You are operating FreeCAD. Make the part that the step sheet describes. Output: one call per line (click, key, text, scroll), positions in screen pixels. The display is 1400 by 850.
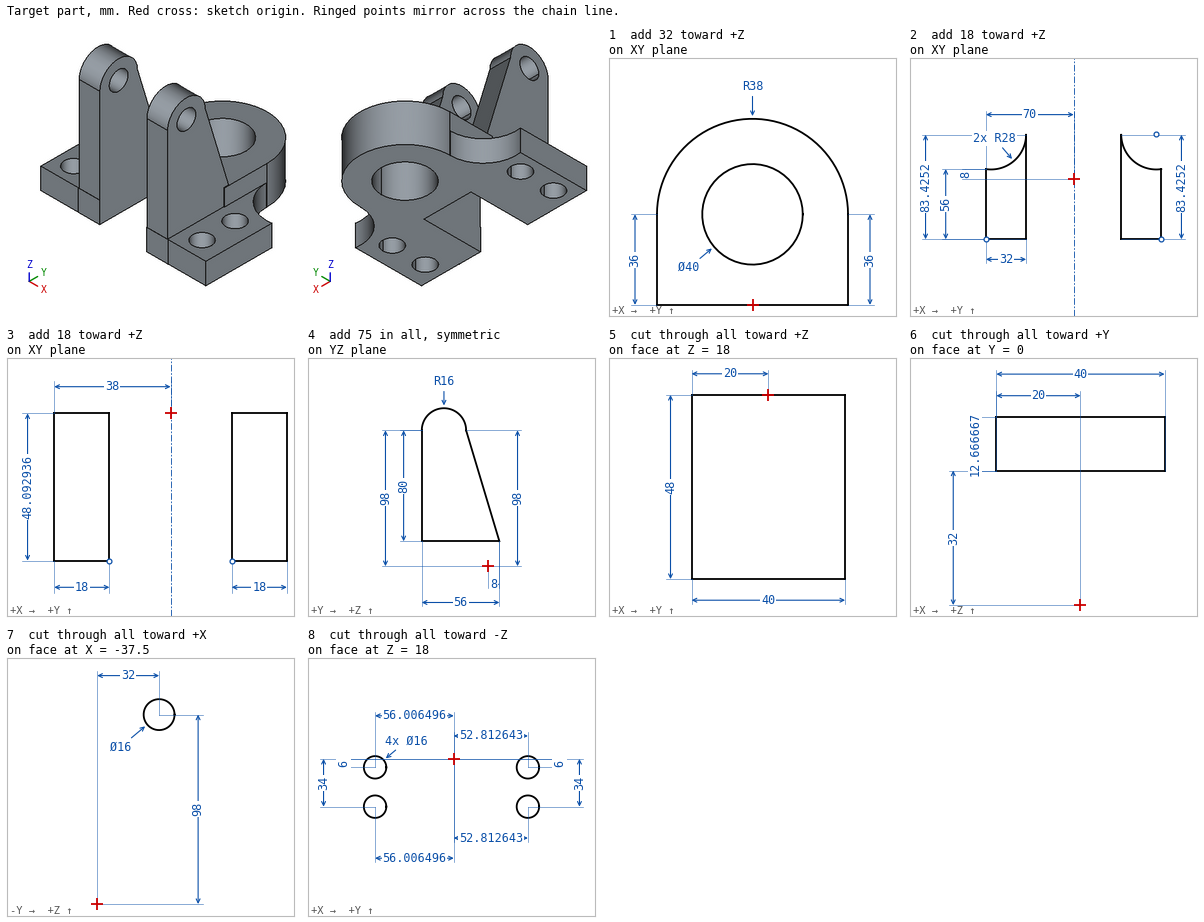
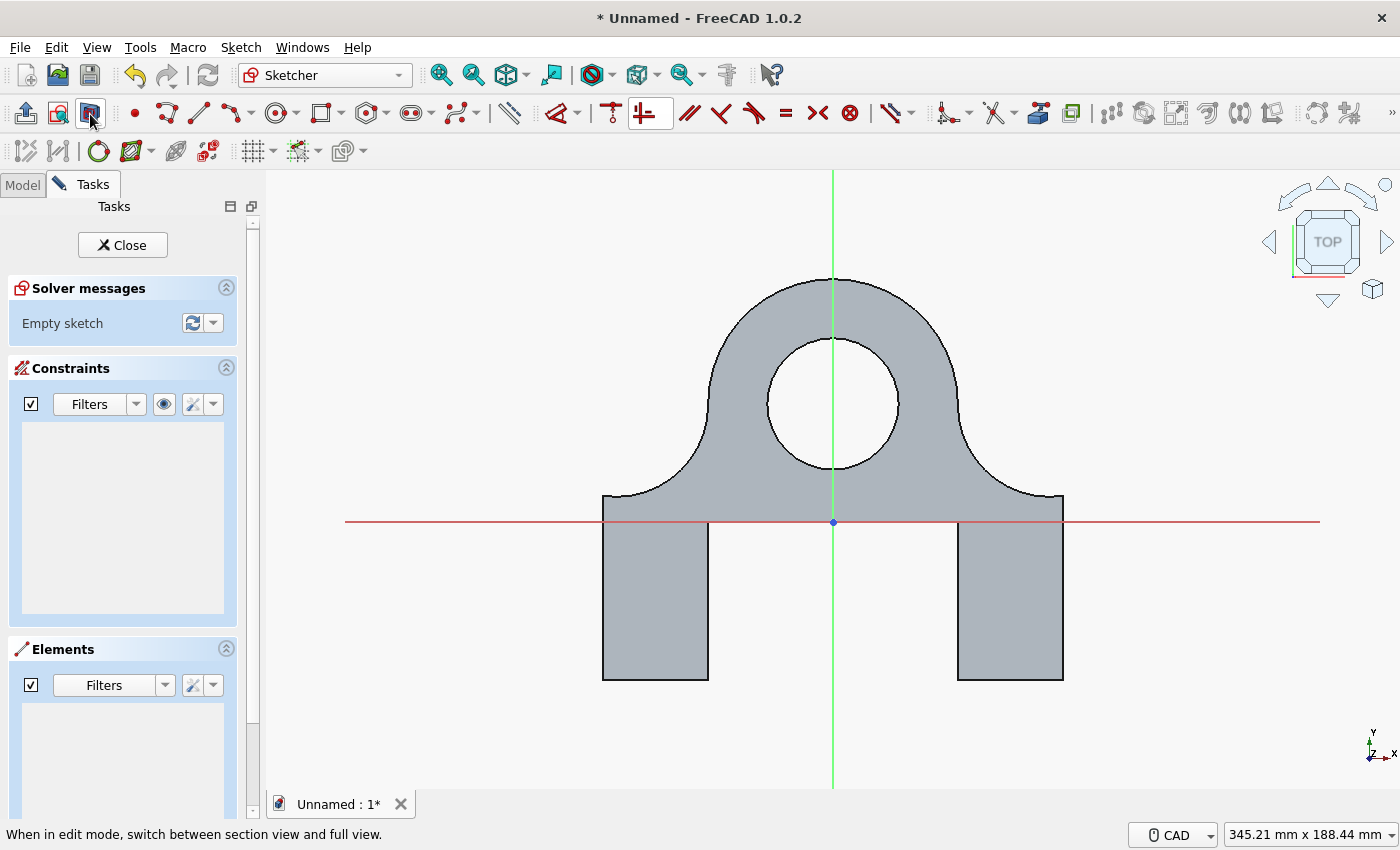
scroll(873, 672, up, 5)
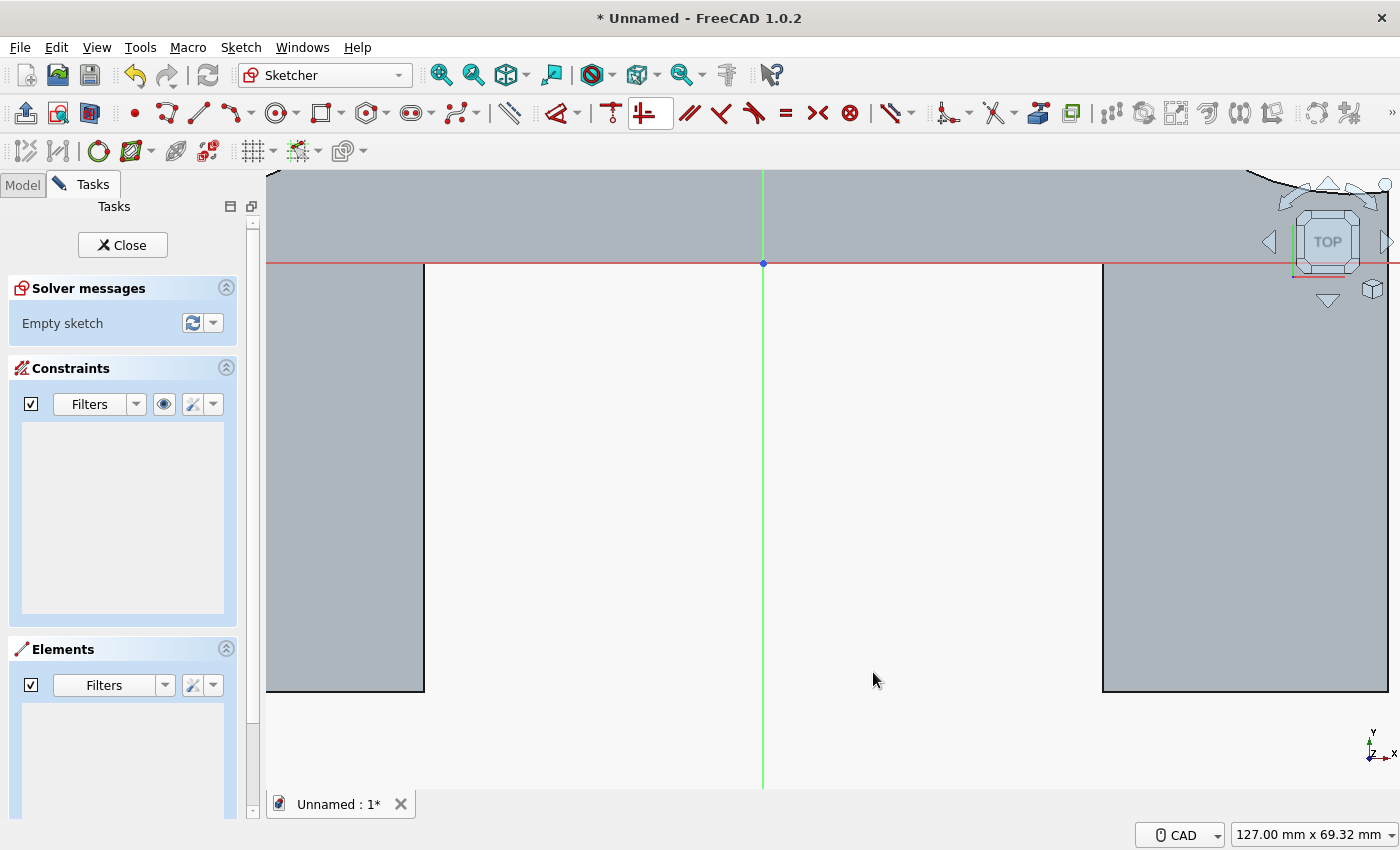
click(322, 114)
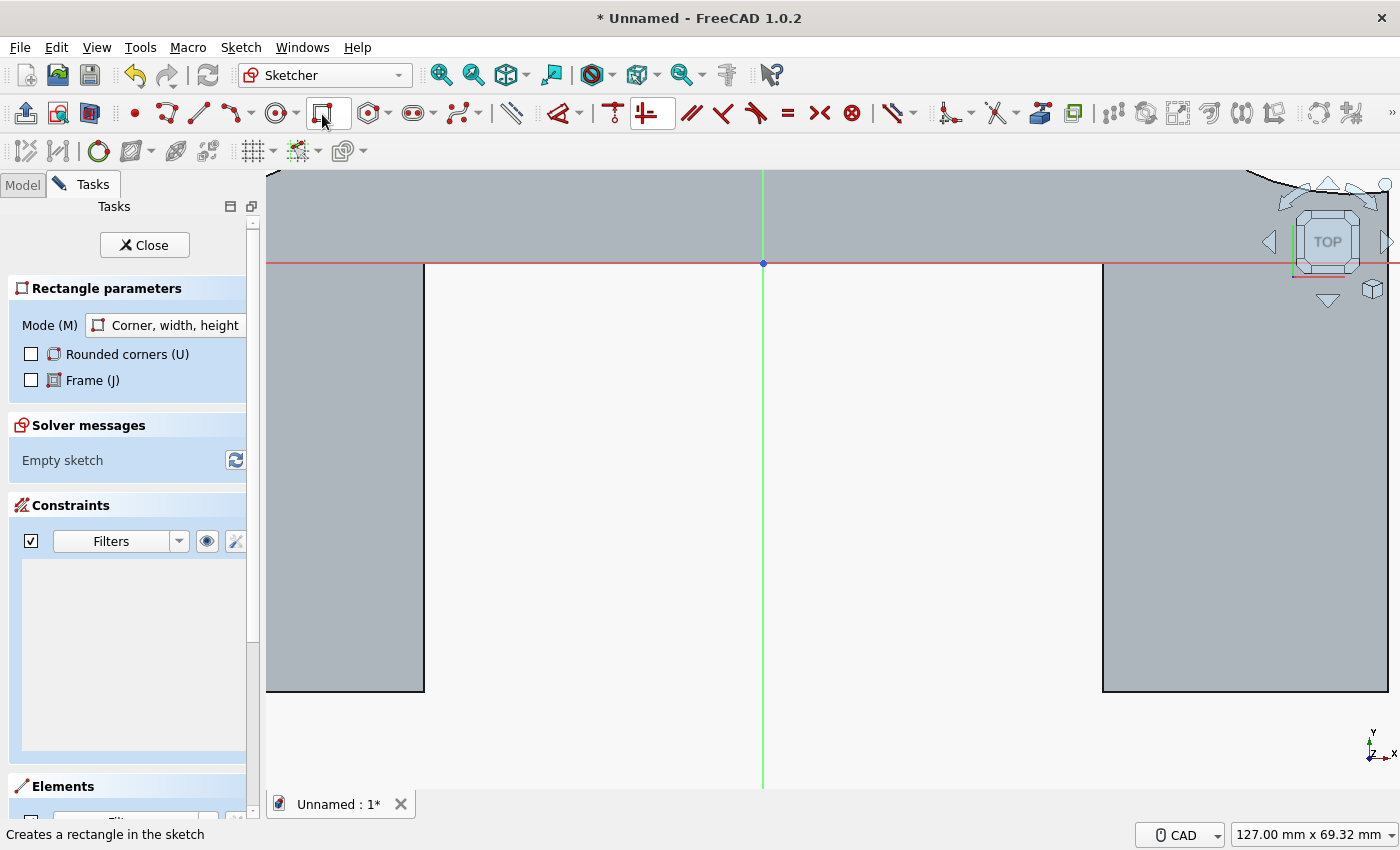
click(424, 263)
click(585, 693)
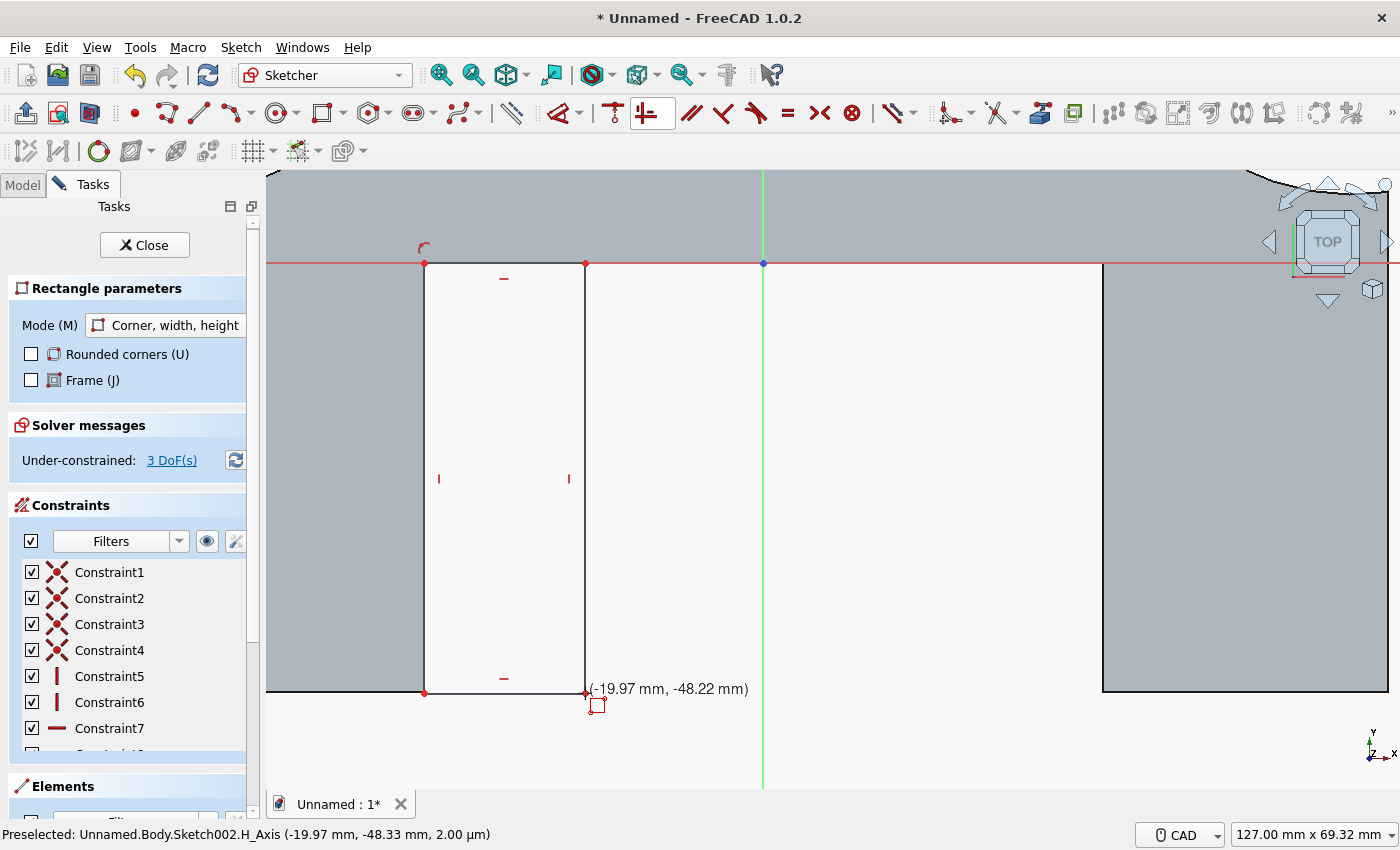
click(942, 263)
click(1103, 693)
key(Escape)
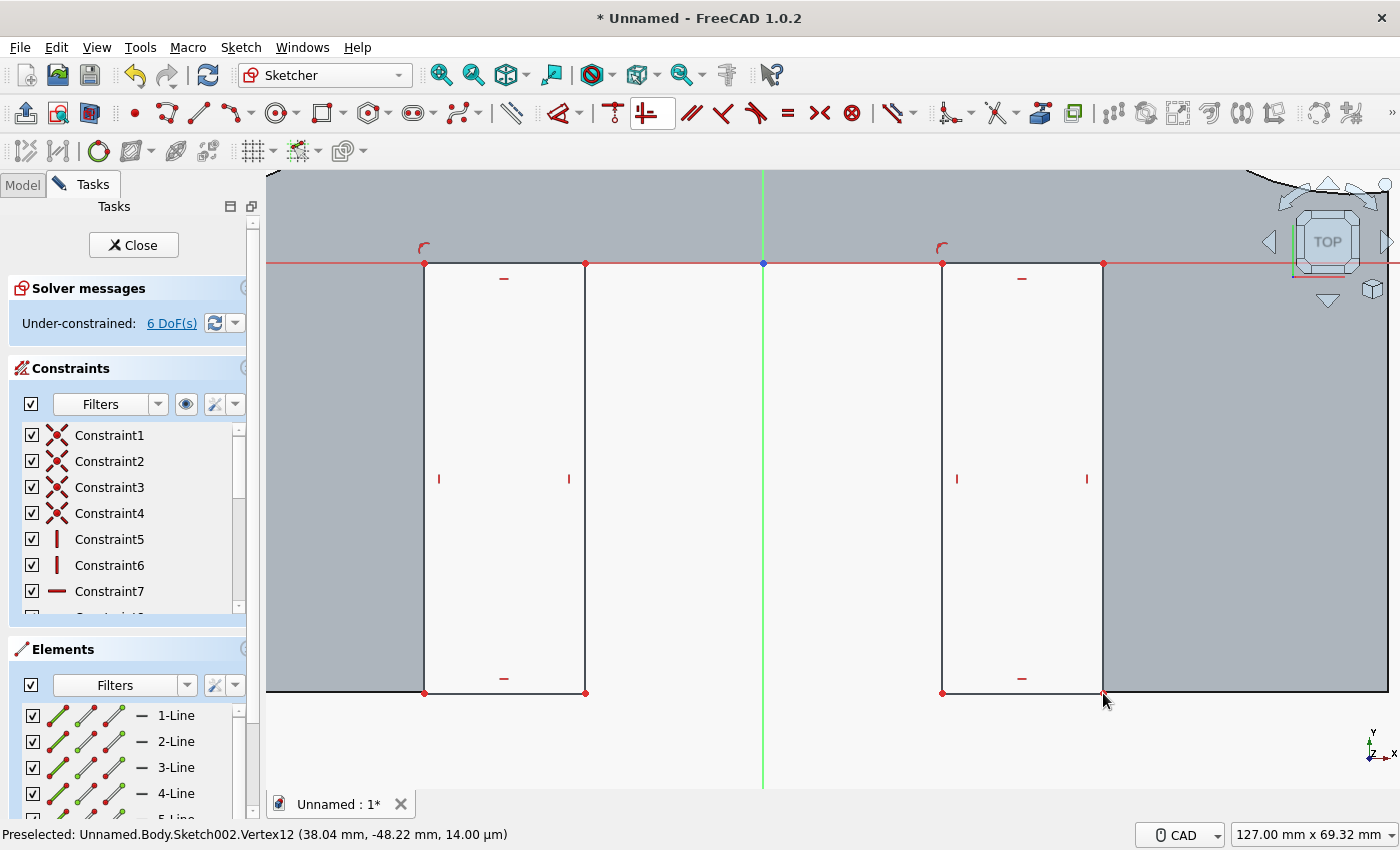
click(585, 694)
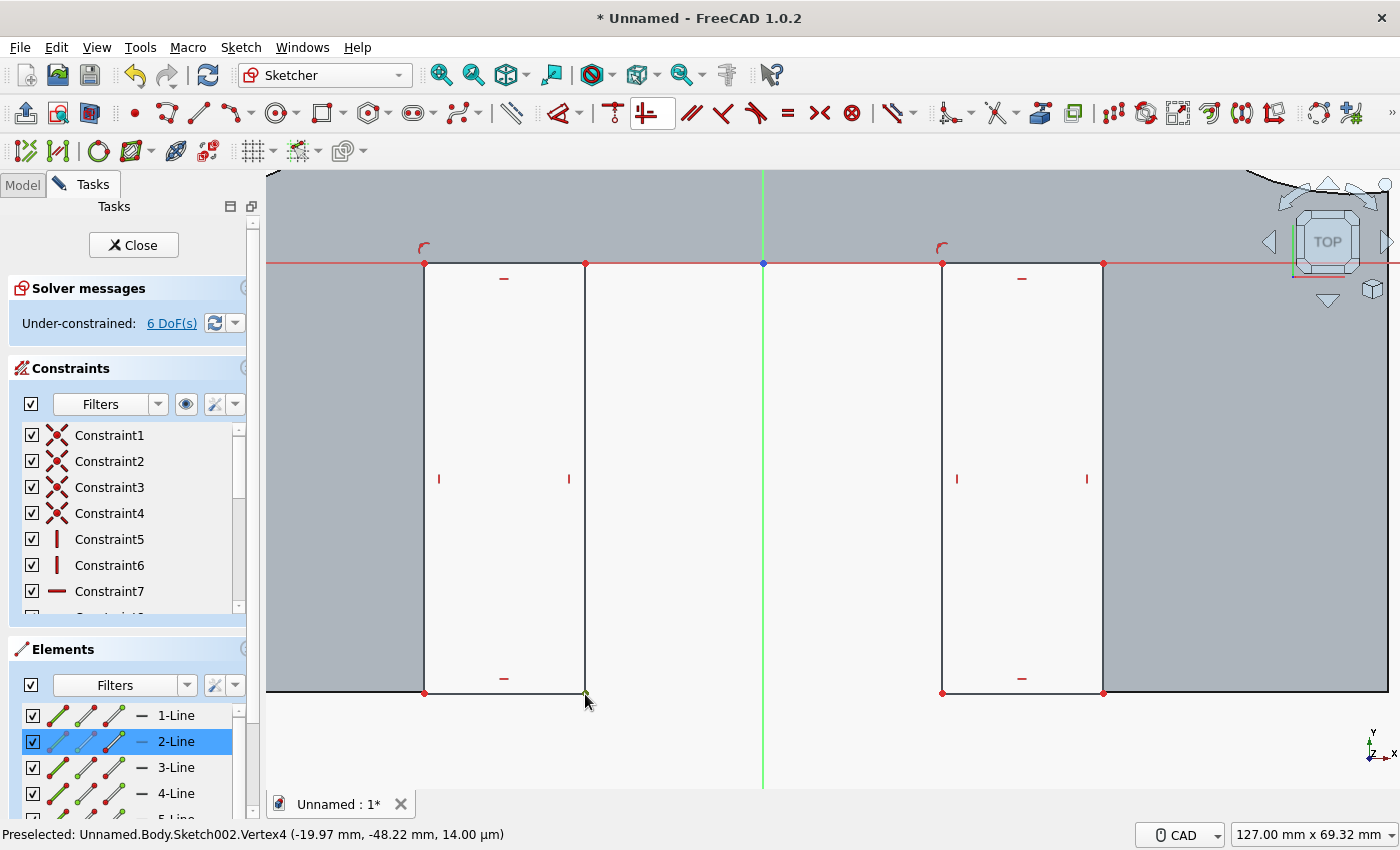
click(942, 694)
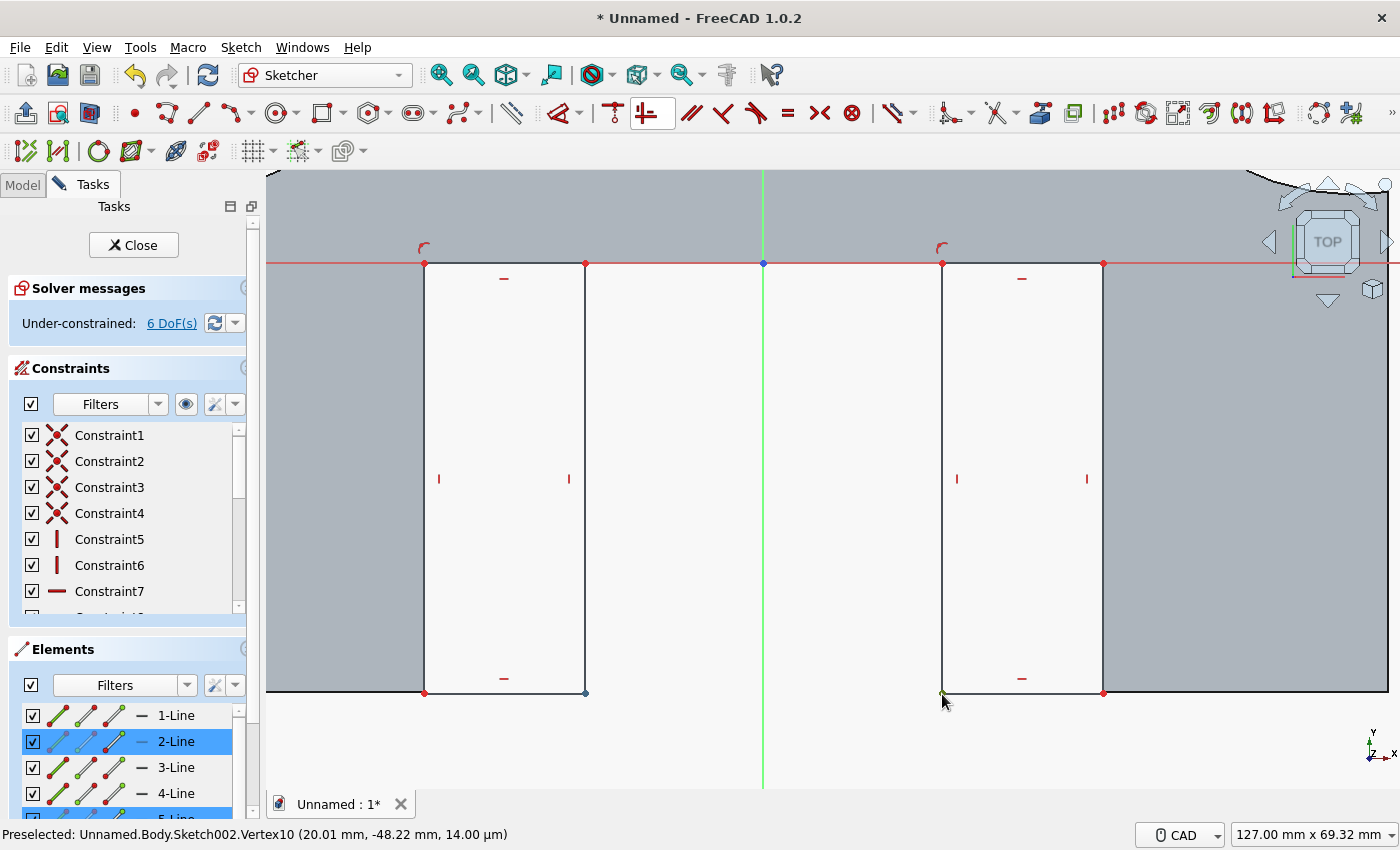
click(763, 721)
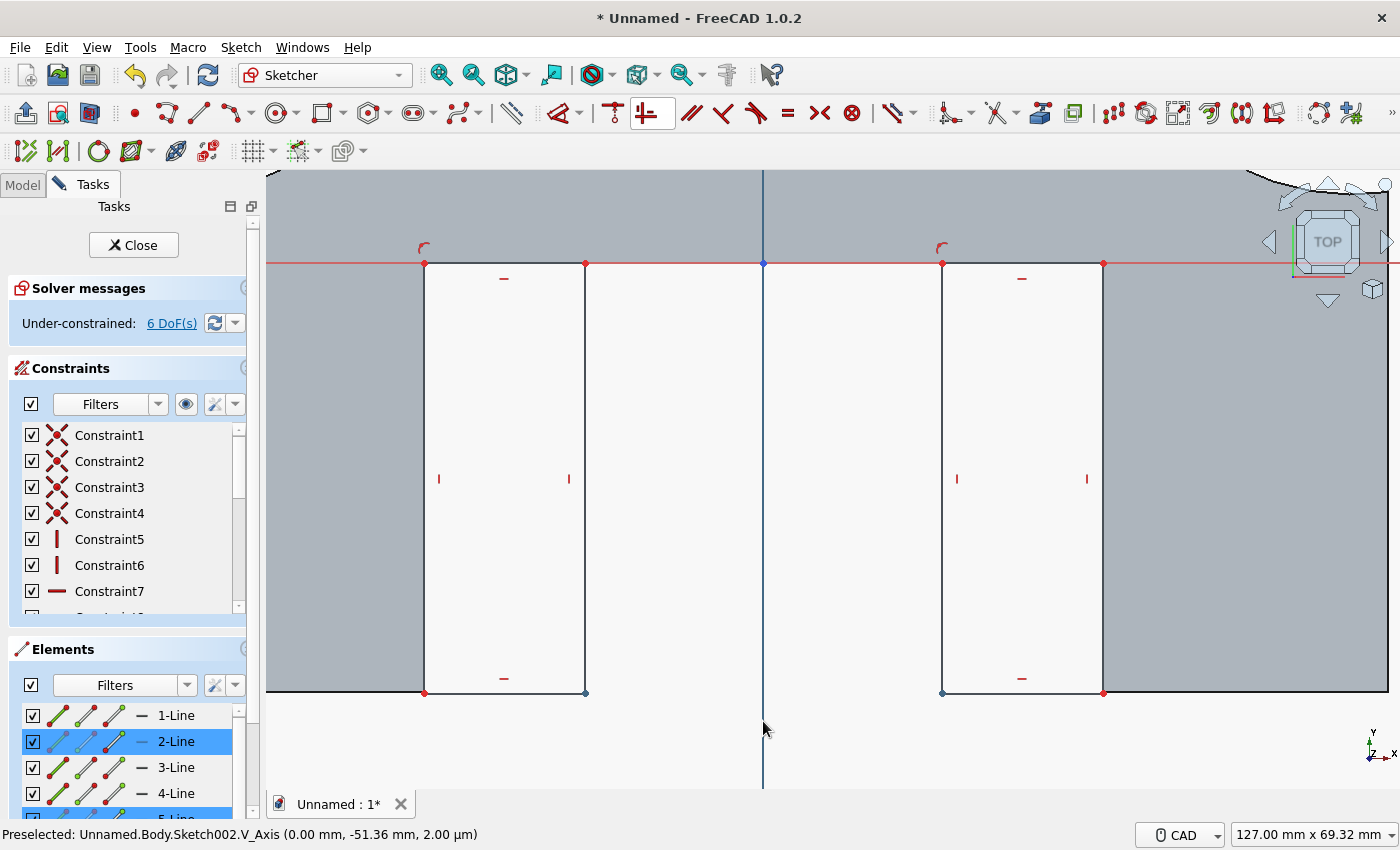
click(820, 114)